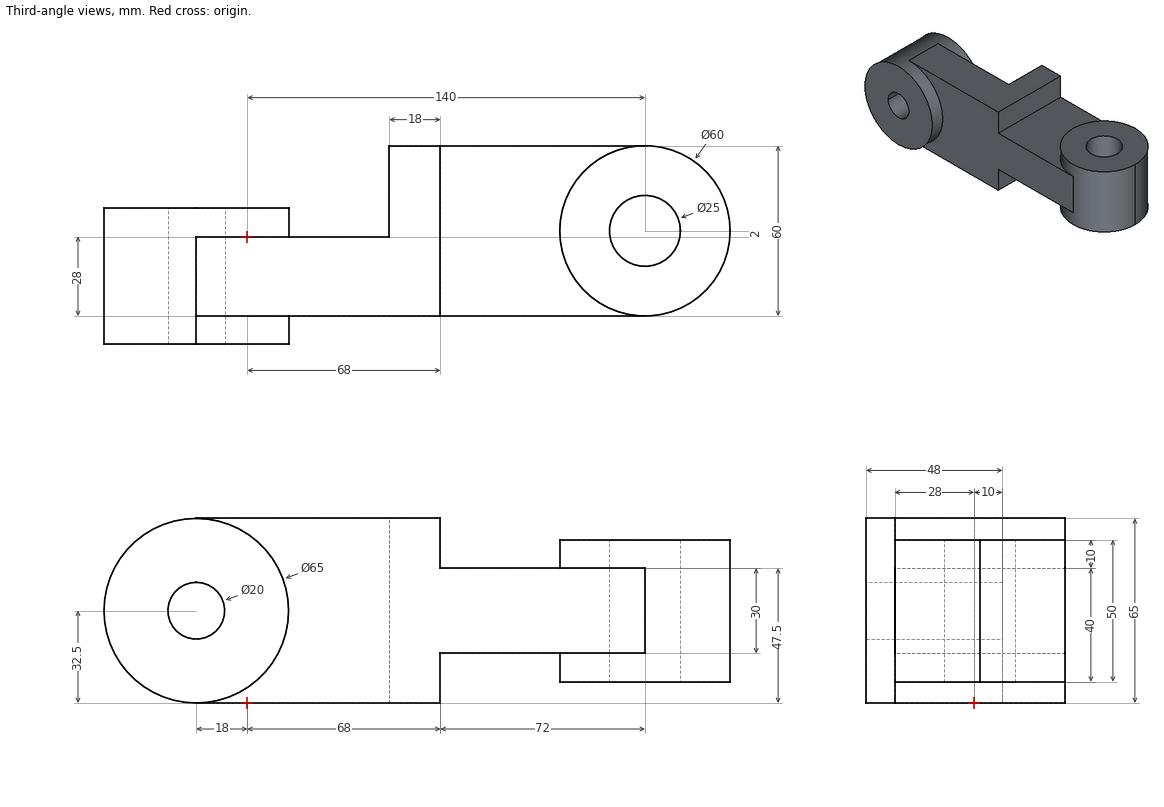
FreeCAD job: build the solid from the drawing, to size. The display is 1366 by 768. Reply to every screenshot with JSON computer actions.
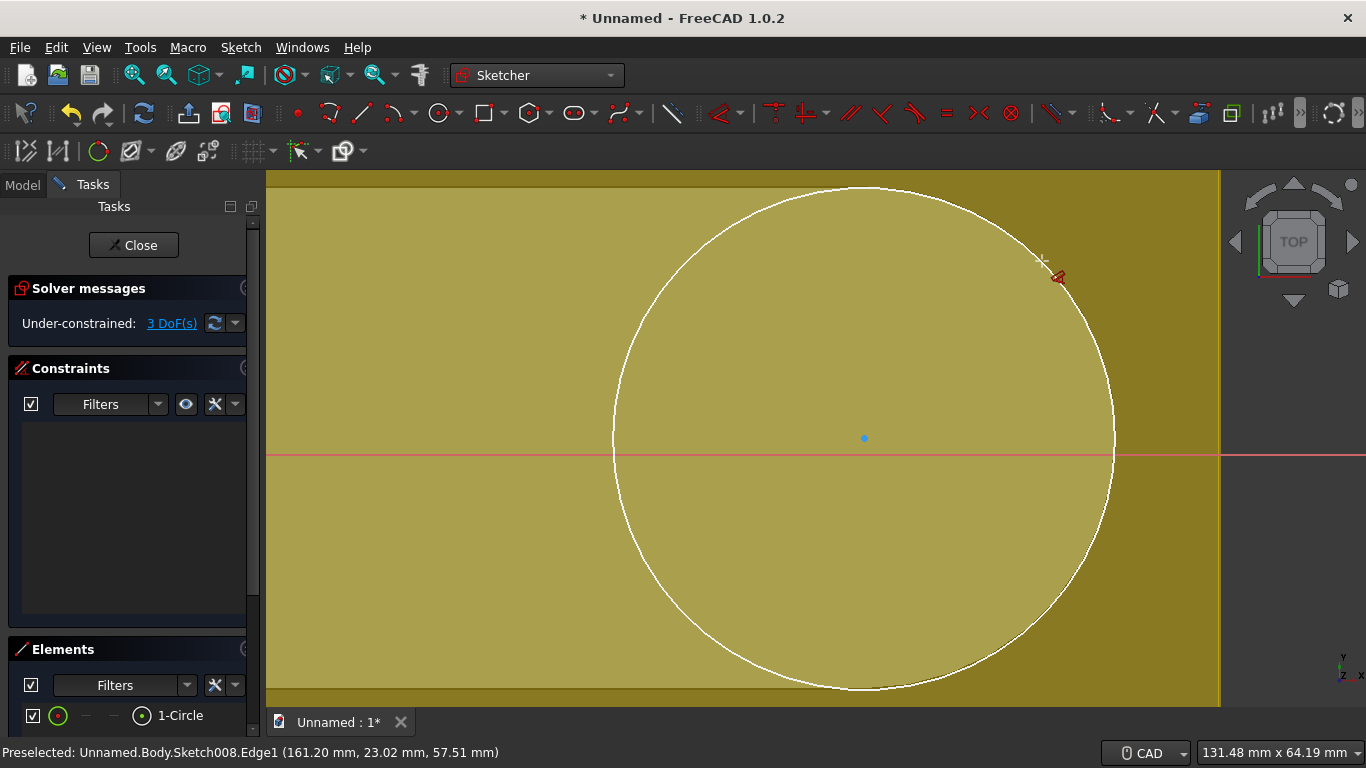
{"action": "left_click", "coordinate": [1041, 261]}
{"action": "left_click", "coordinate": [1064, 238]}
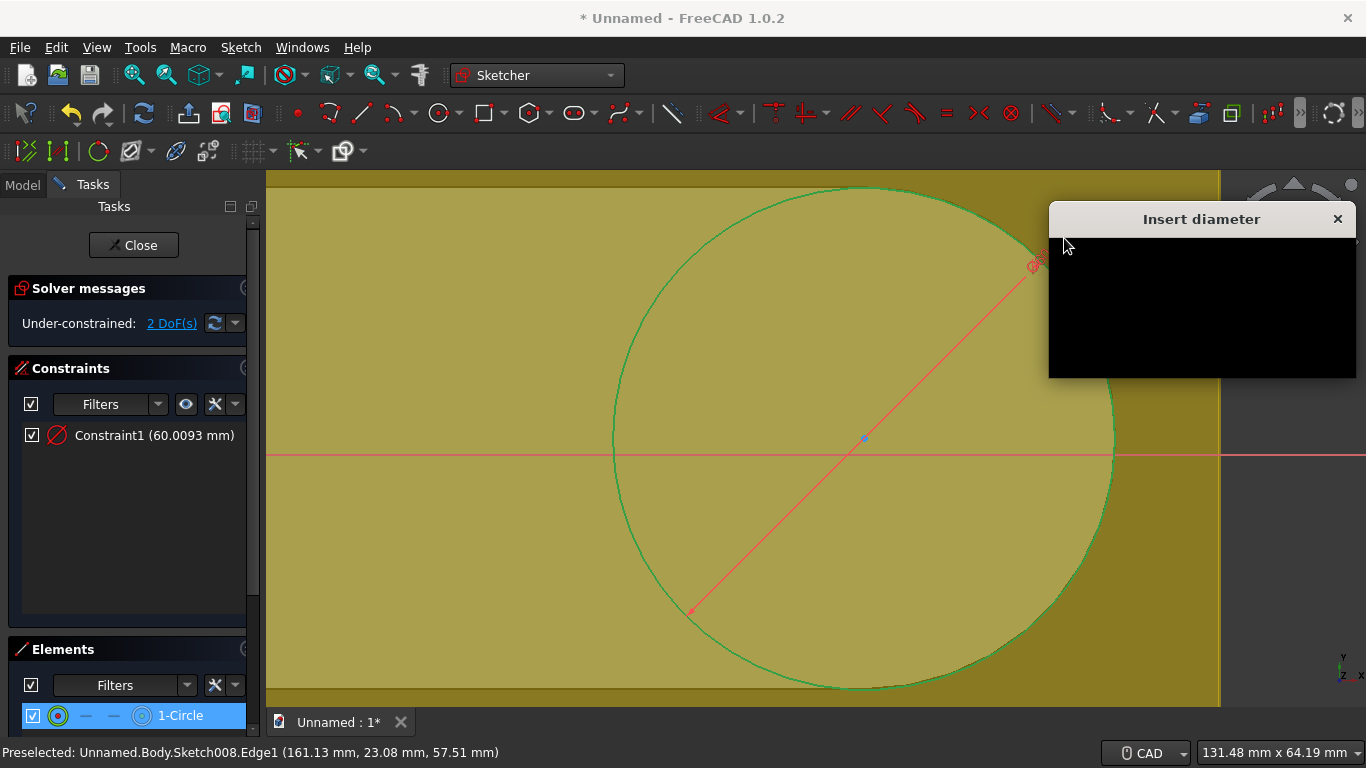
{"action": "type", "text": "60"}
{"action": "key", "text": "Return"}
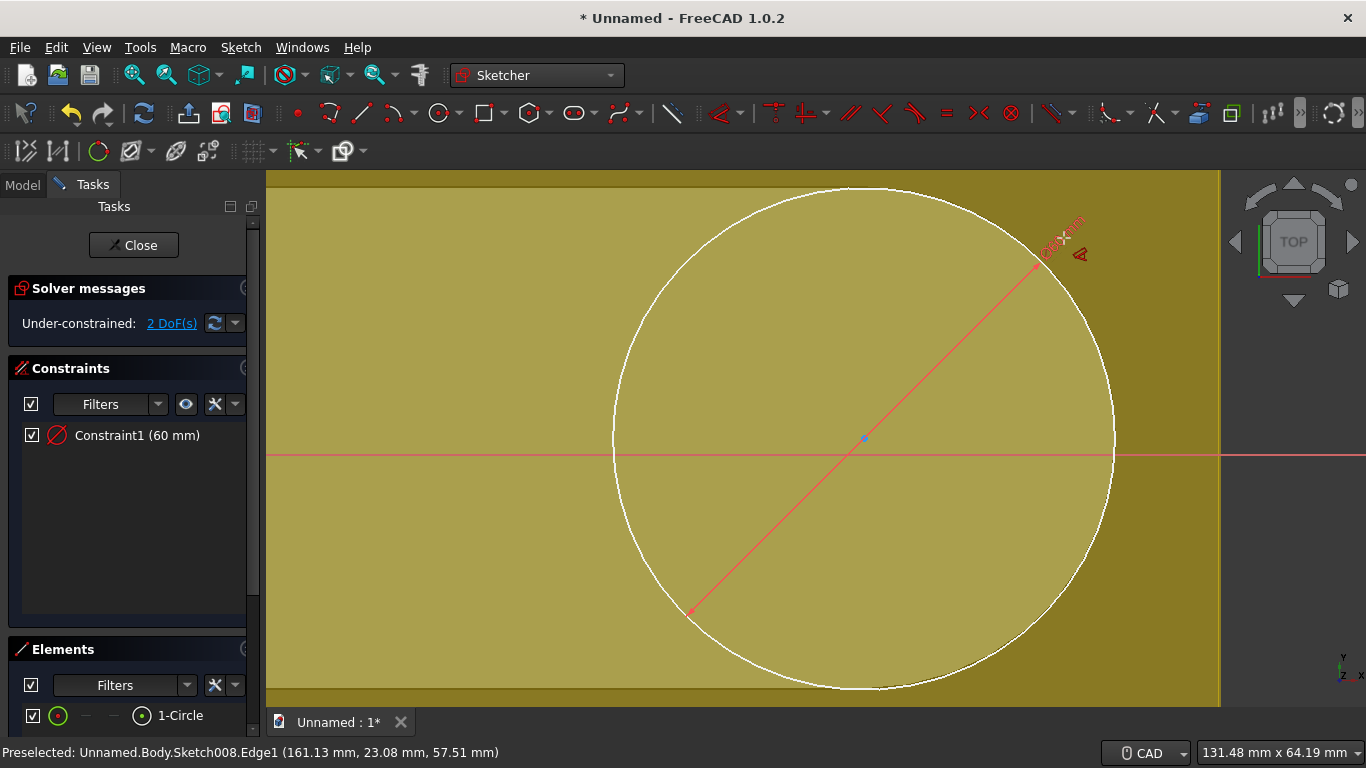
{"action": "scroll", "coordinate": [864, 439], "scroll_direction": "up", "scroll_amount": 5}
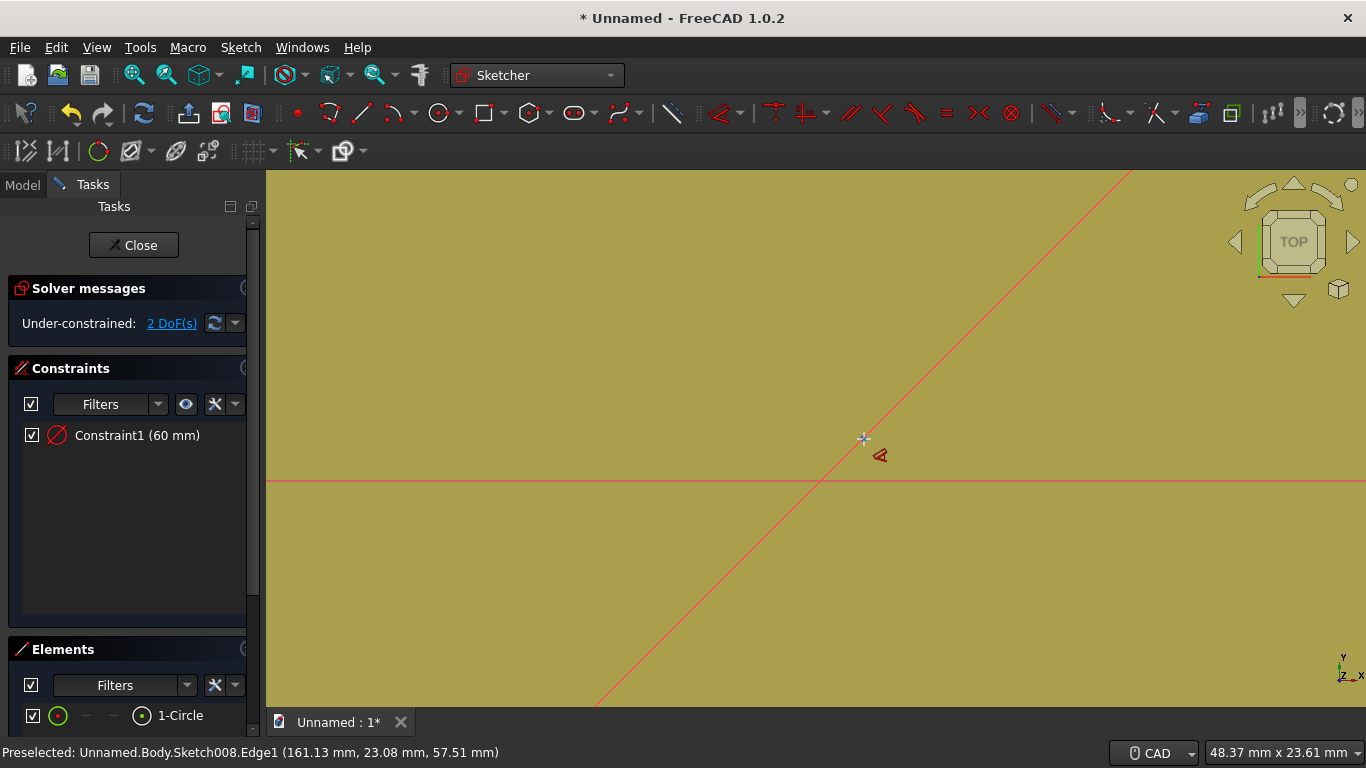
{"action": "left_click", "coordinate": [863, 438]}
{"action": "left_click", "coordinate": [897, 460]}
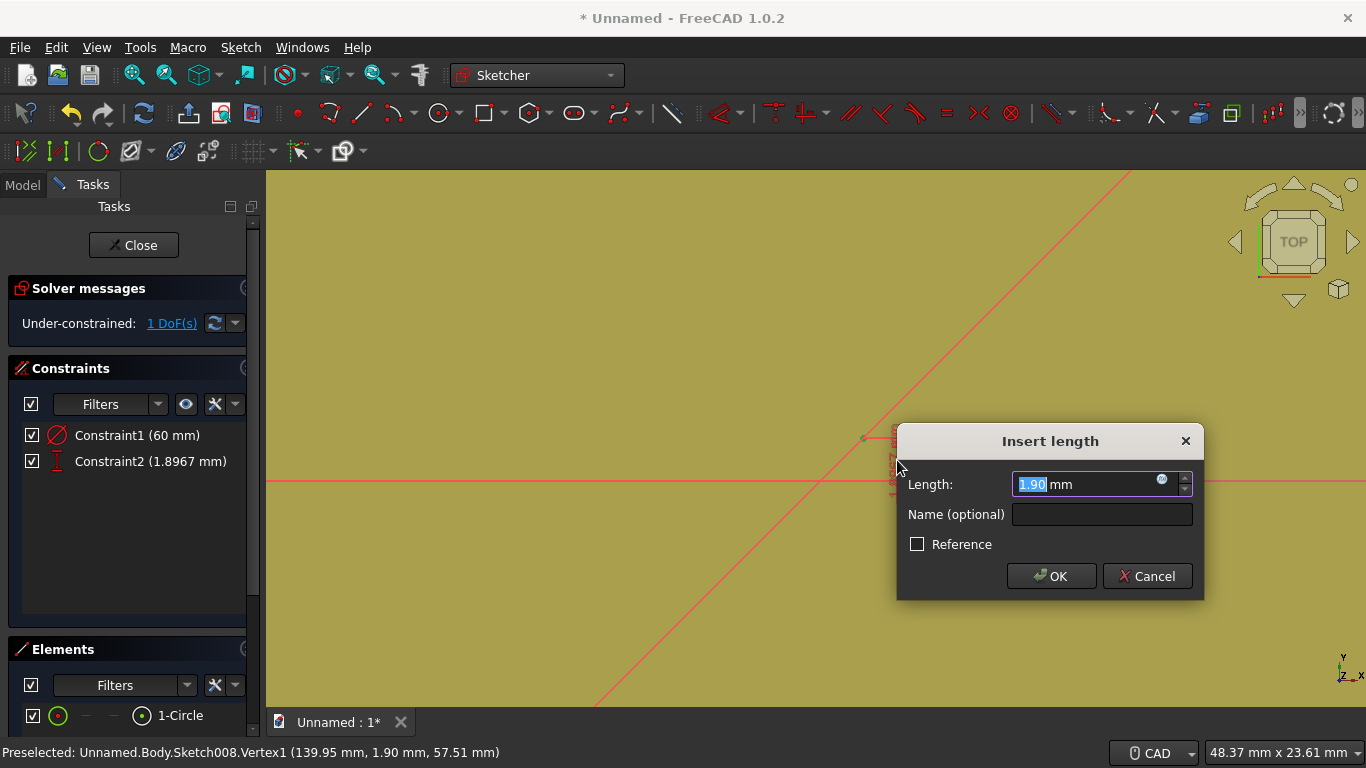
{"action": "type", "text": "2"}
{"action": "key", "text": "Return"}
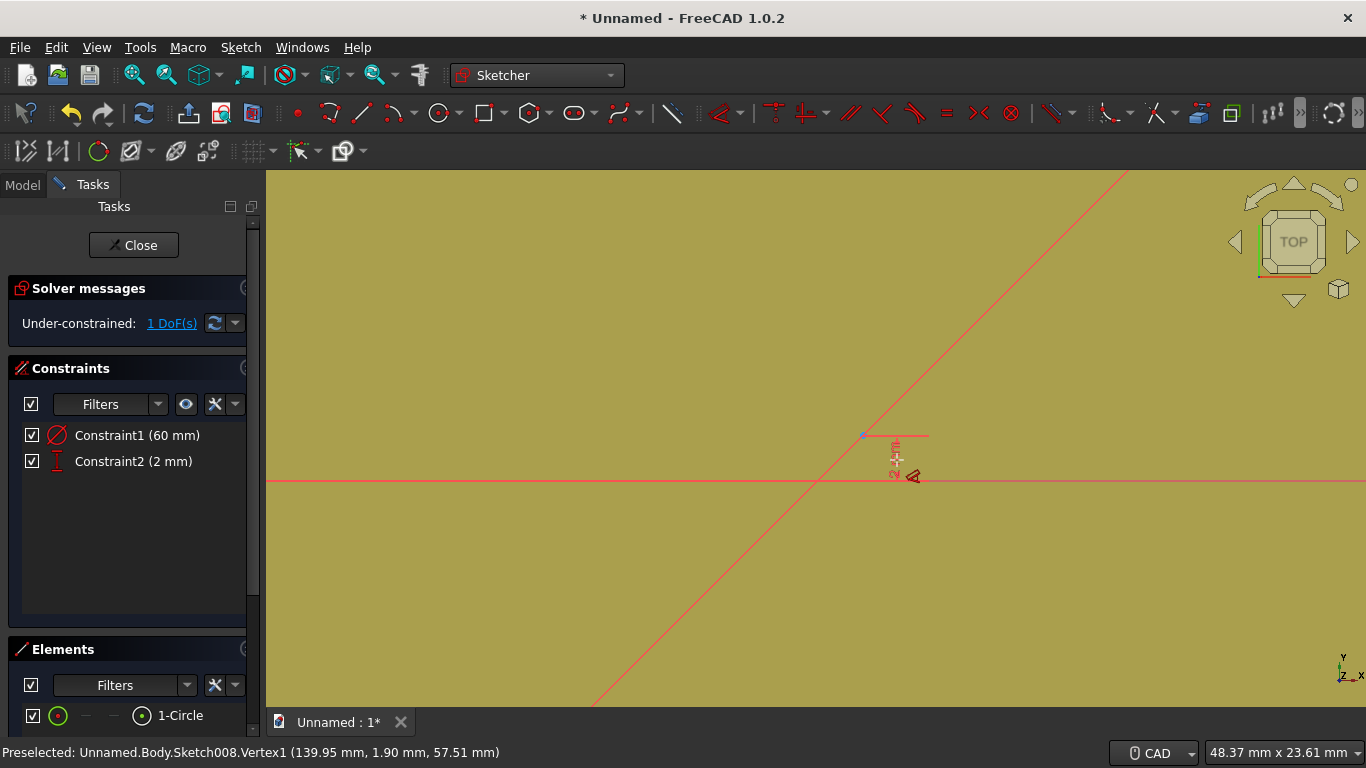
{"action": "scroll", "coordinate": [709, 439], "scroll_direction": "down", "scroll_amount": 7}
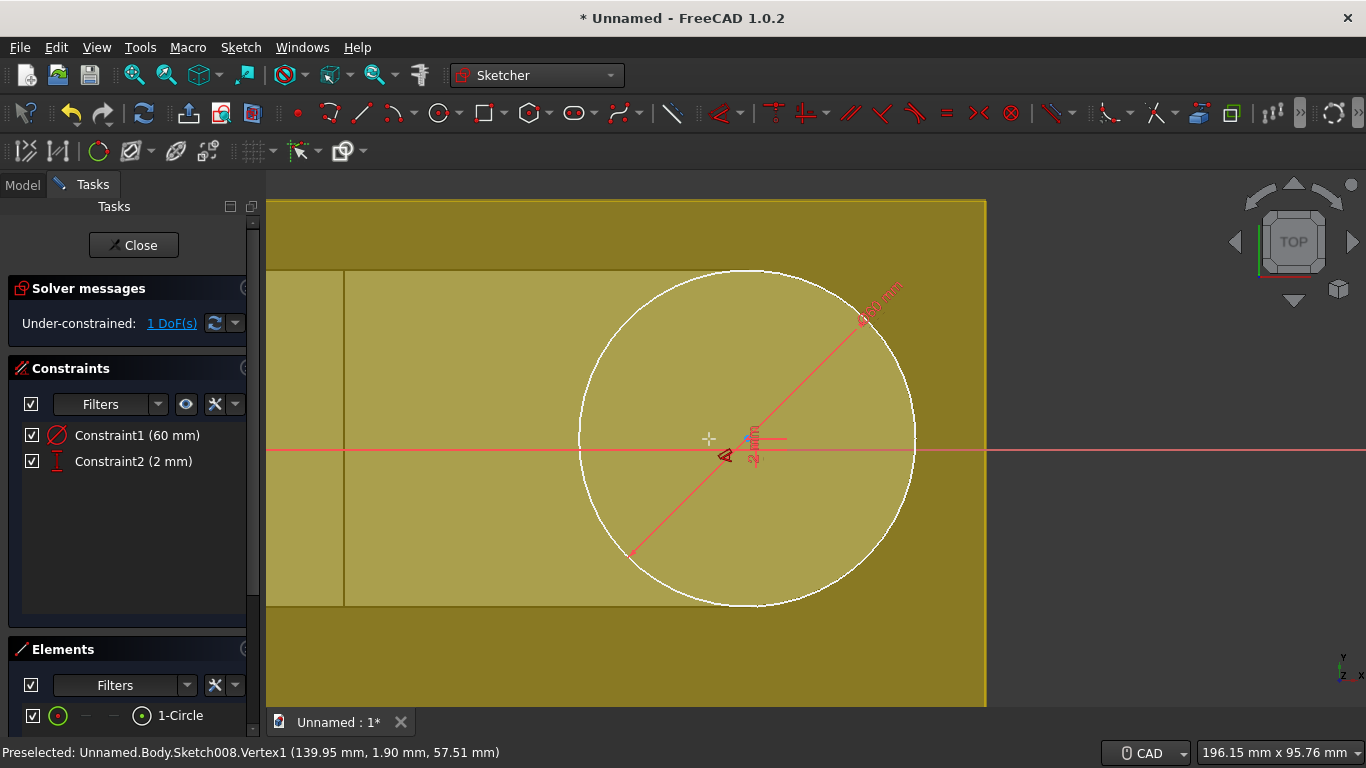
{"action": "left_click", "coordinate": [747, 439]}
{"action": "left_click", "coordinate": [521, 484]}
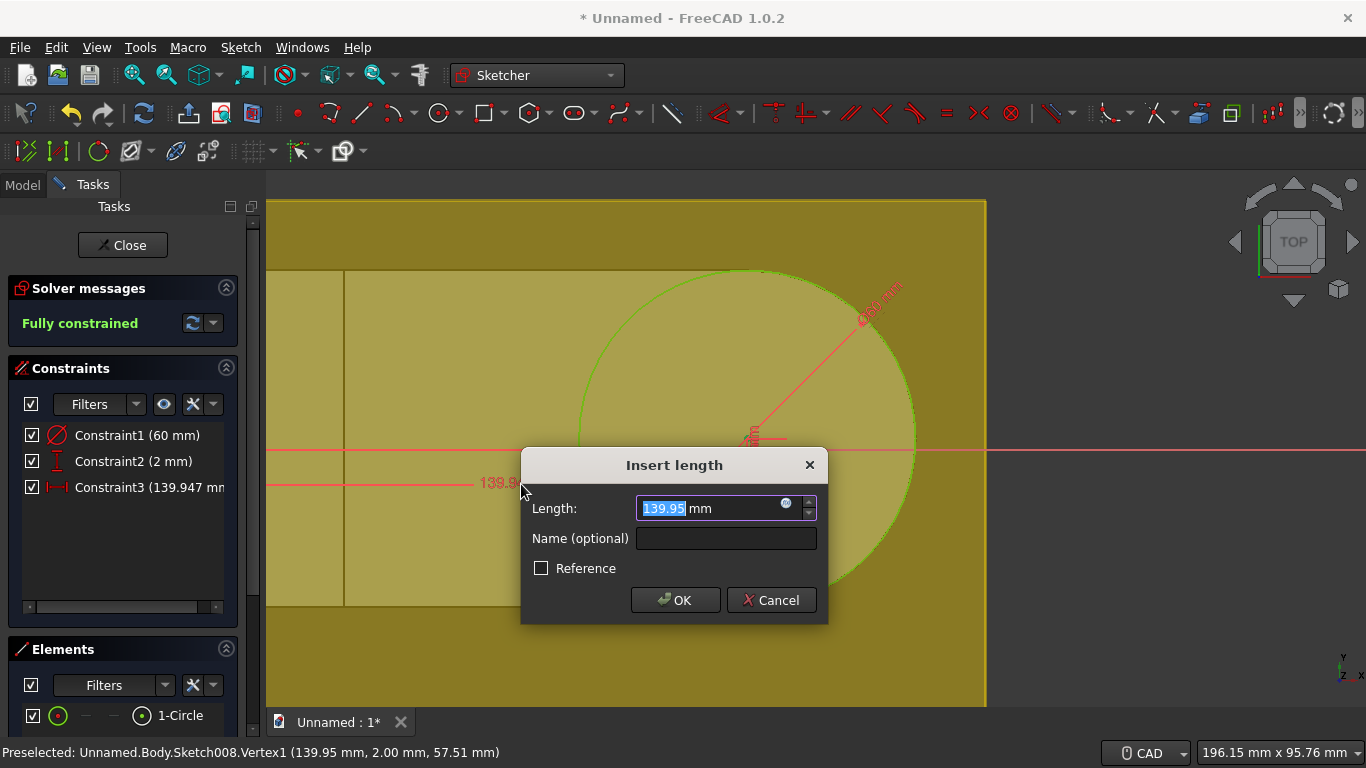
{"action": "type", "text": "140"}
{"action": "key", "text": "Return"}
{"action": "key", "text": "Escape"}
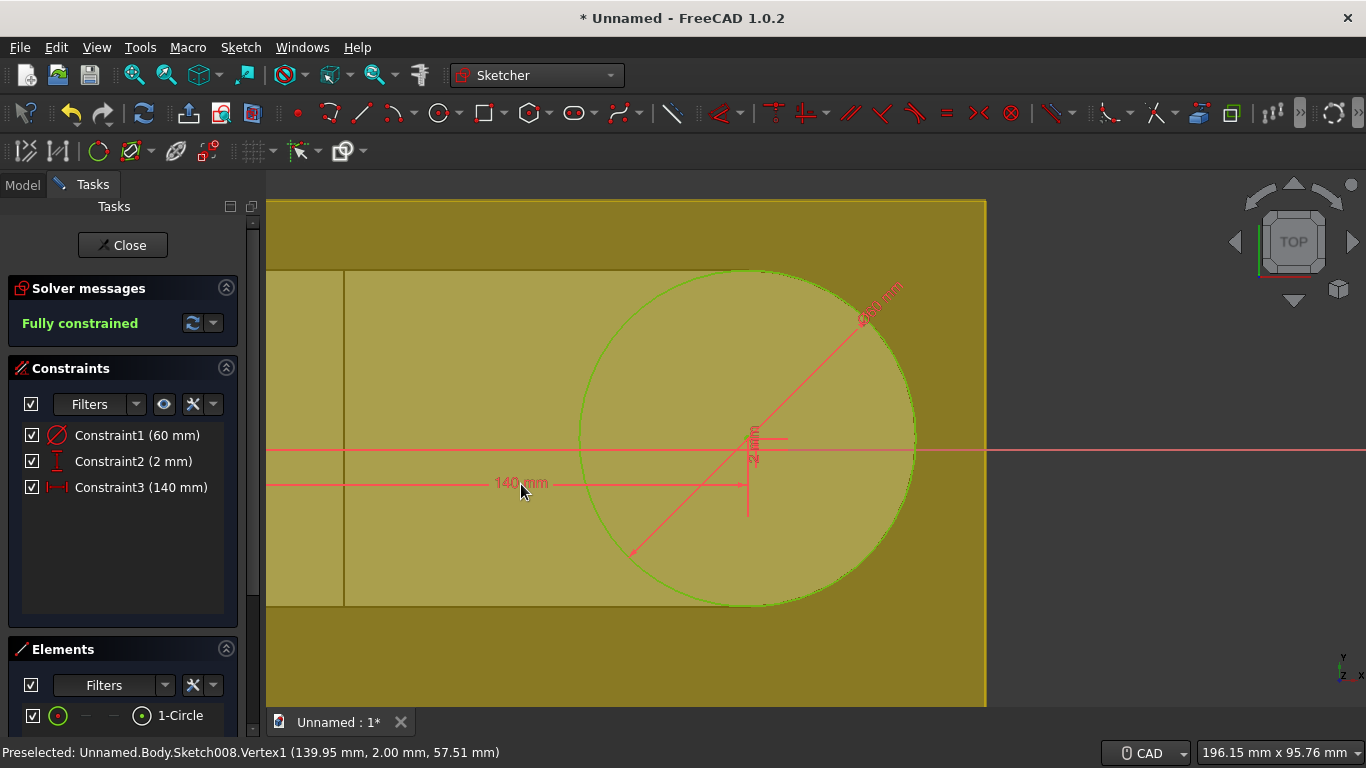
{"action": "left_click", "coordinate": [123, 245]}